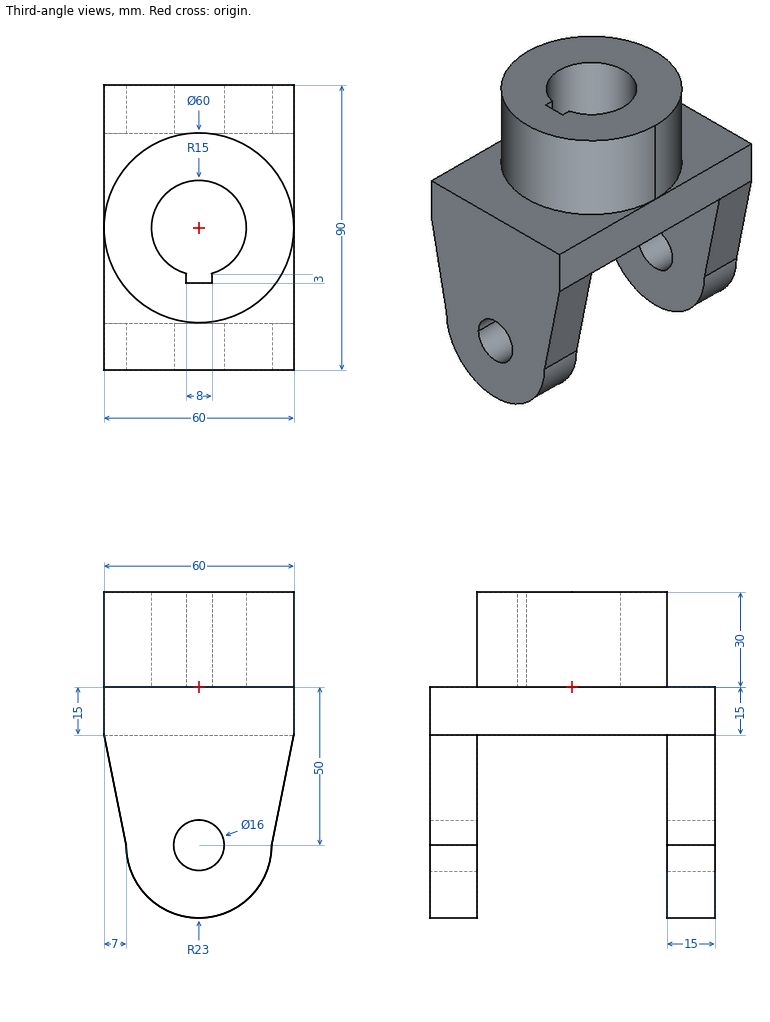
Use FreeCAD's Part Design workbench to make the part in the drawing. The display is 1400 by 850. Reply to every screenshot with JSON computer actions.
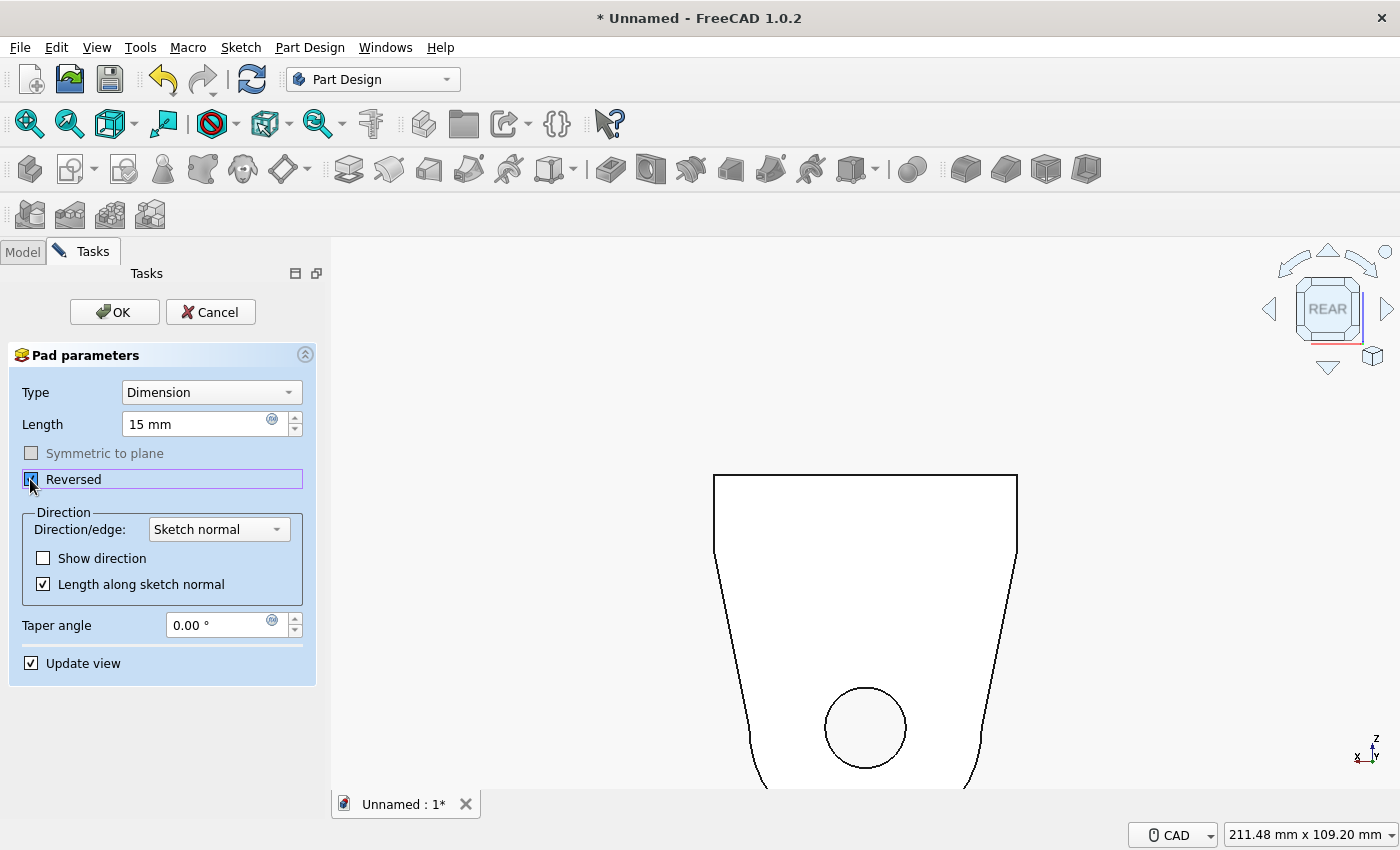
{"action": "left_click", "coordinate": [115, 312]}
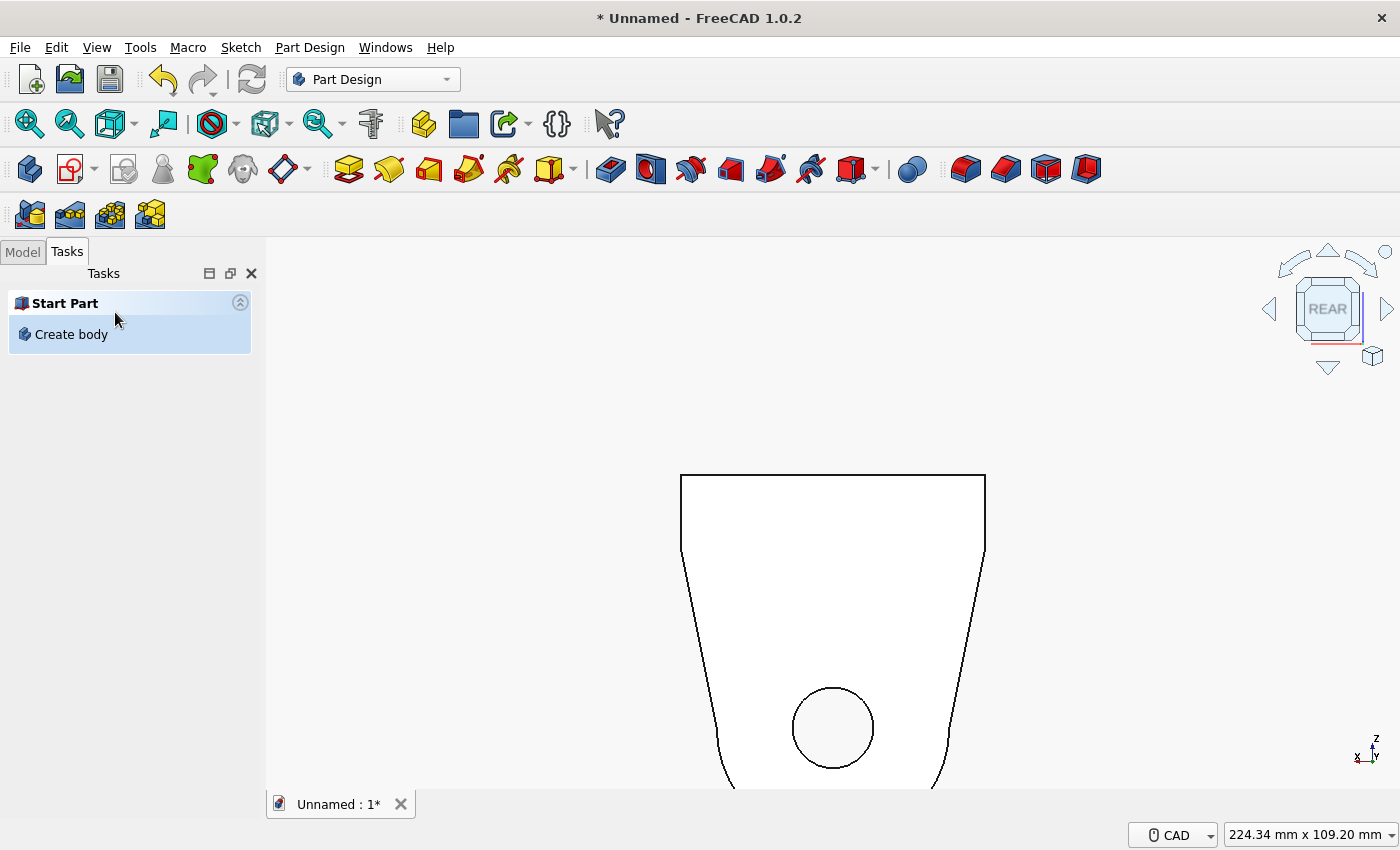
{"action": "left_click", "coordinate": [30, 124]}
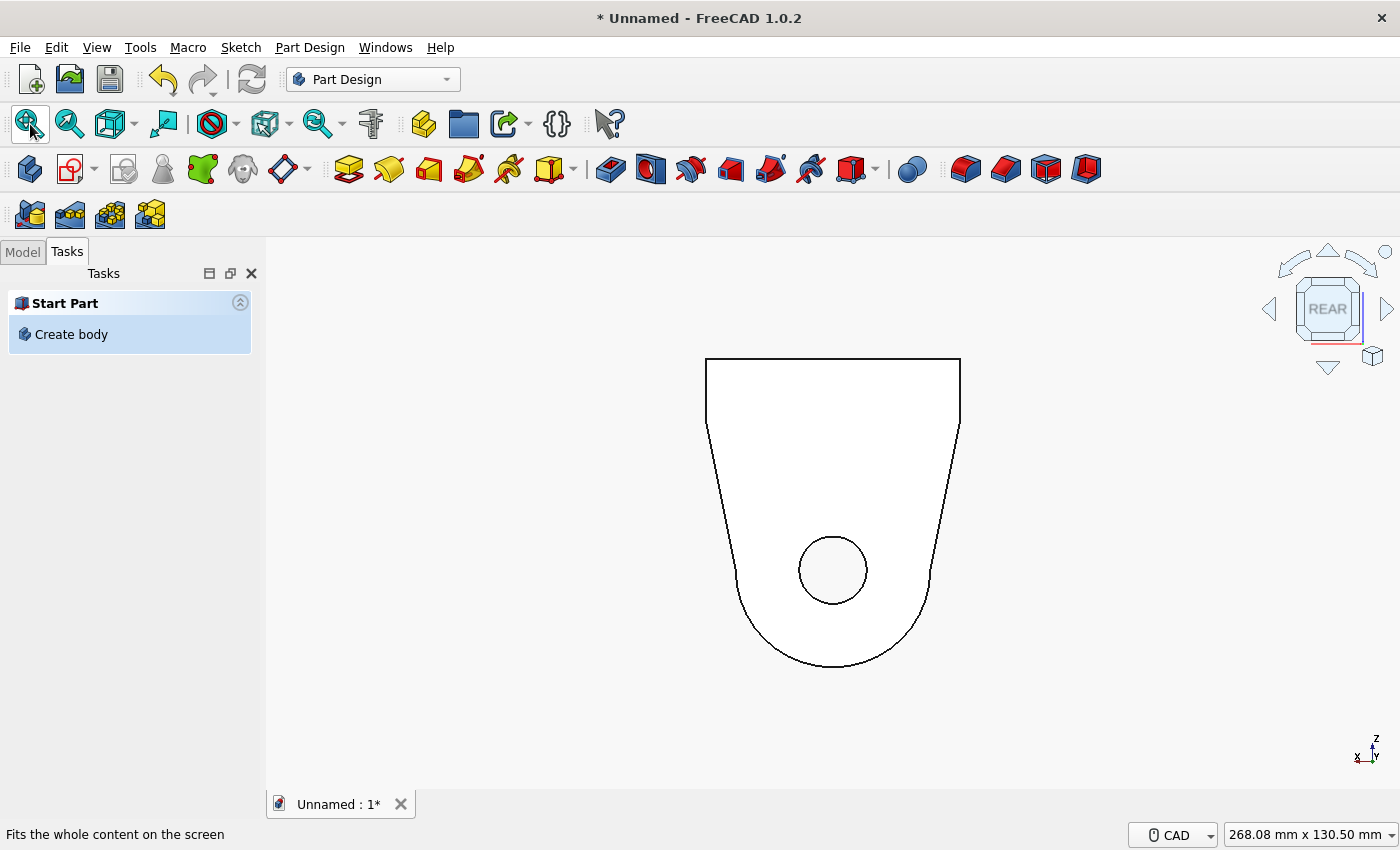
{"action": "left_click", "coordinate": [23, 251]}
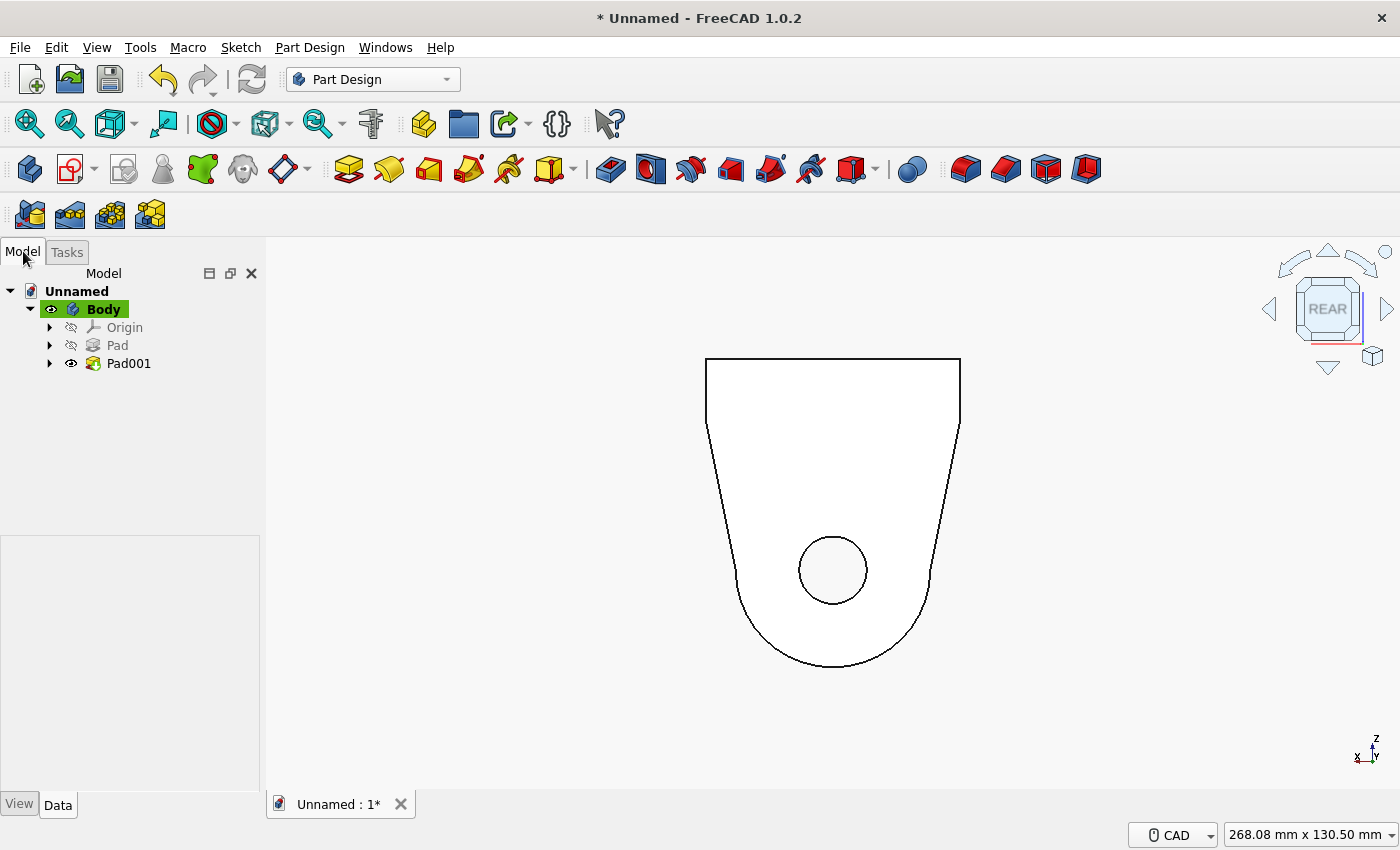
{"action": "left_click", "coordinate": [116, 363]}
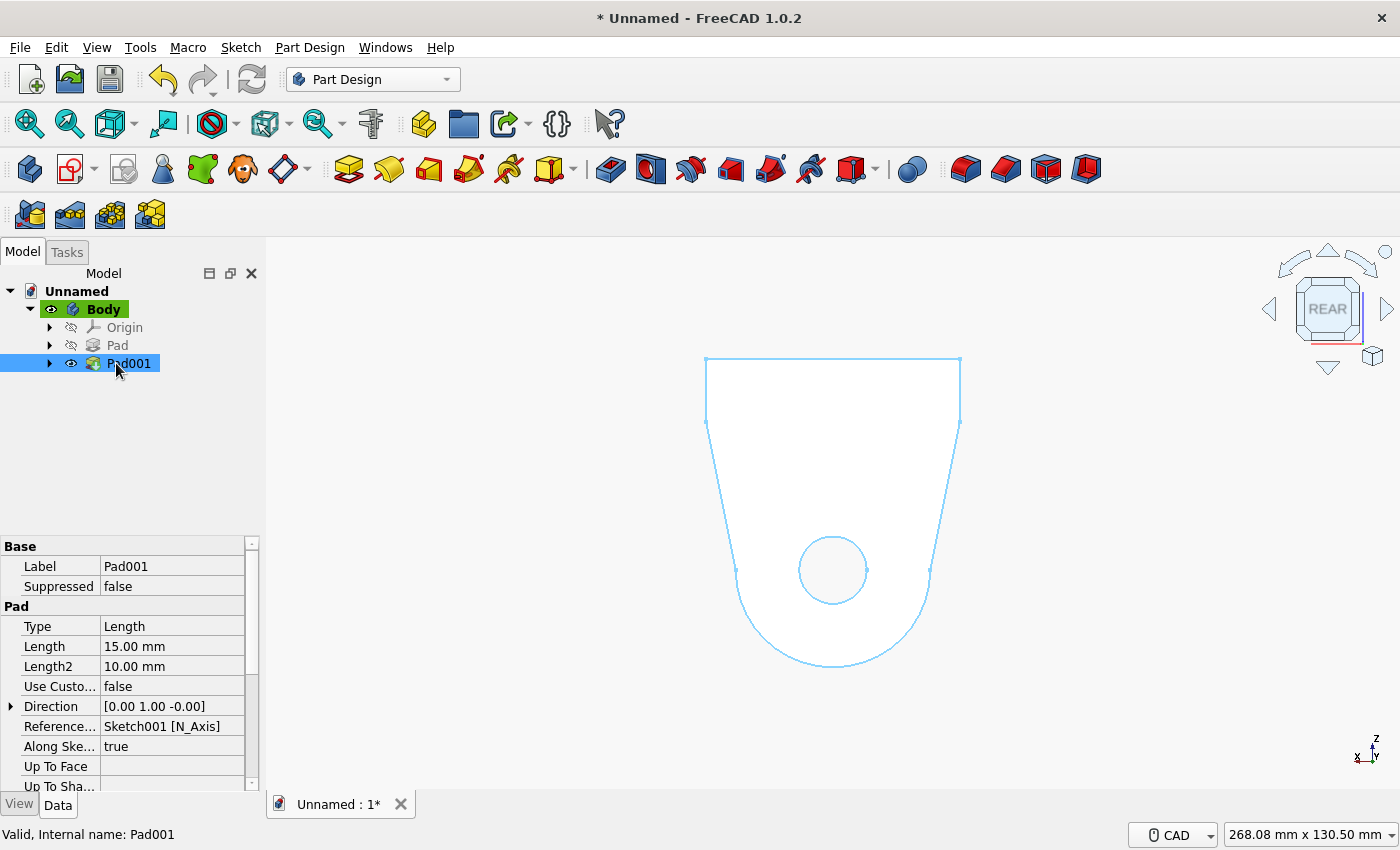
{"action": "left_click", "coordinate": [30, 214]}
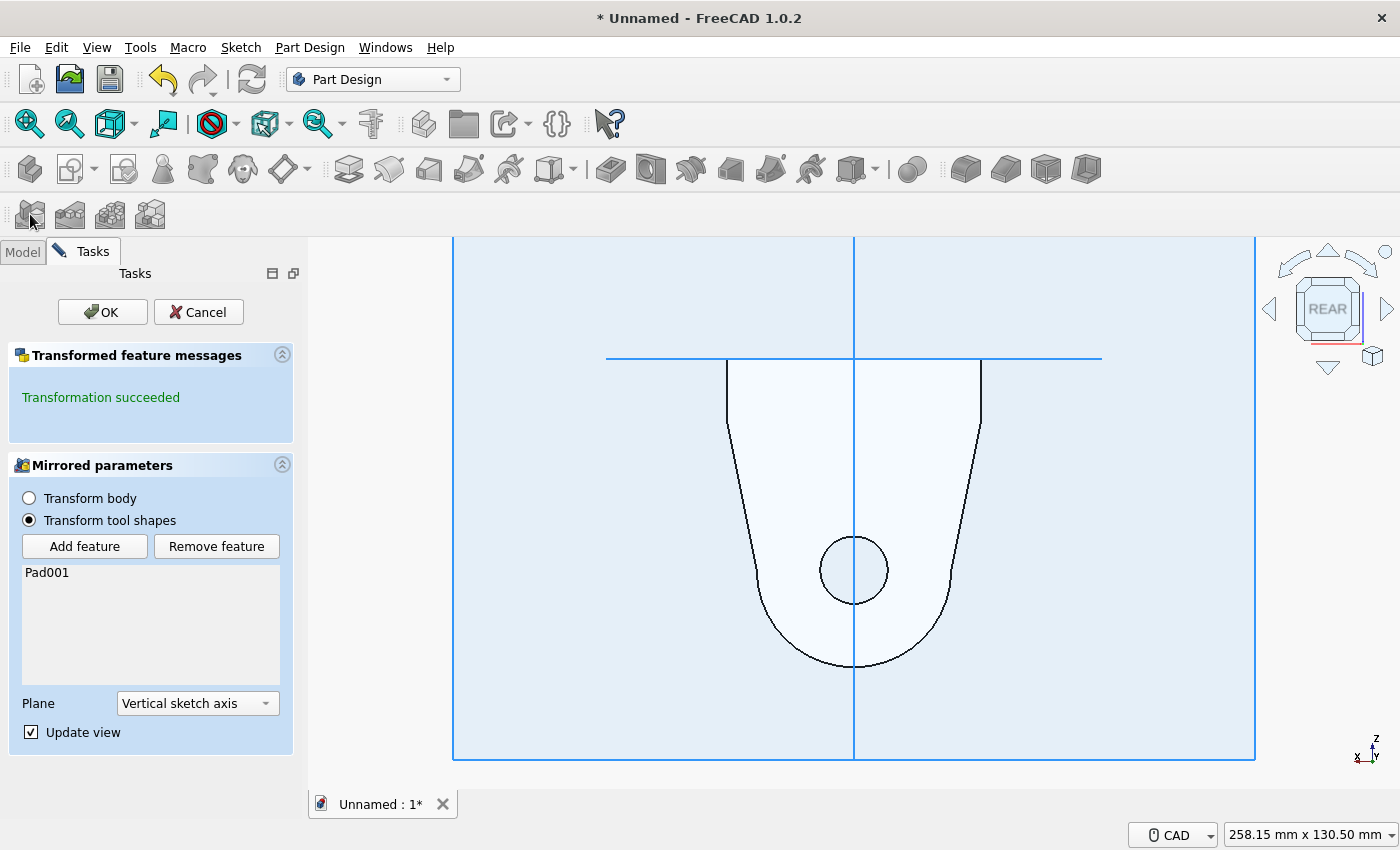
{"action": "left_click", "coordinate": [198, 704]}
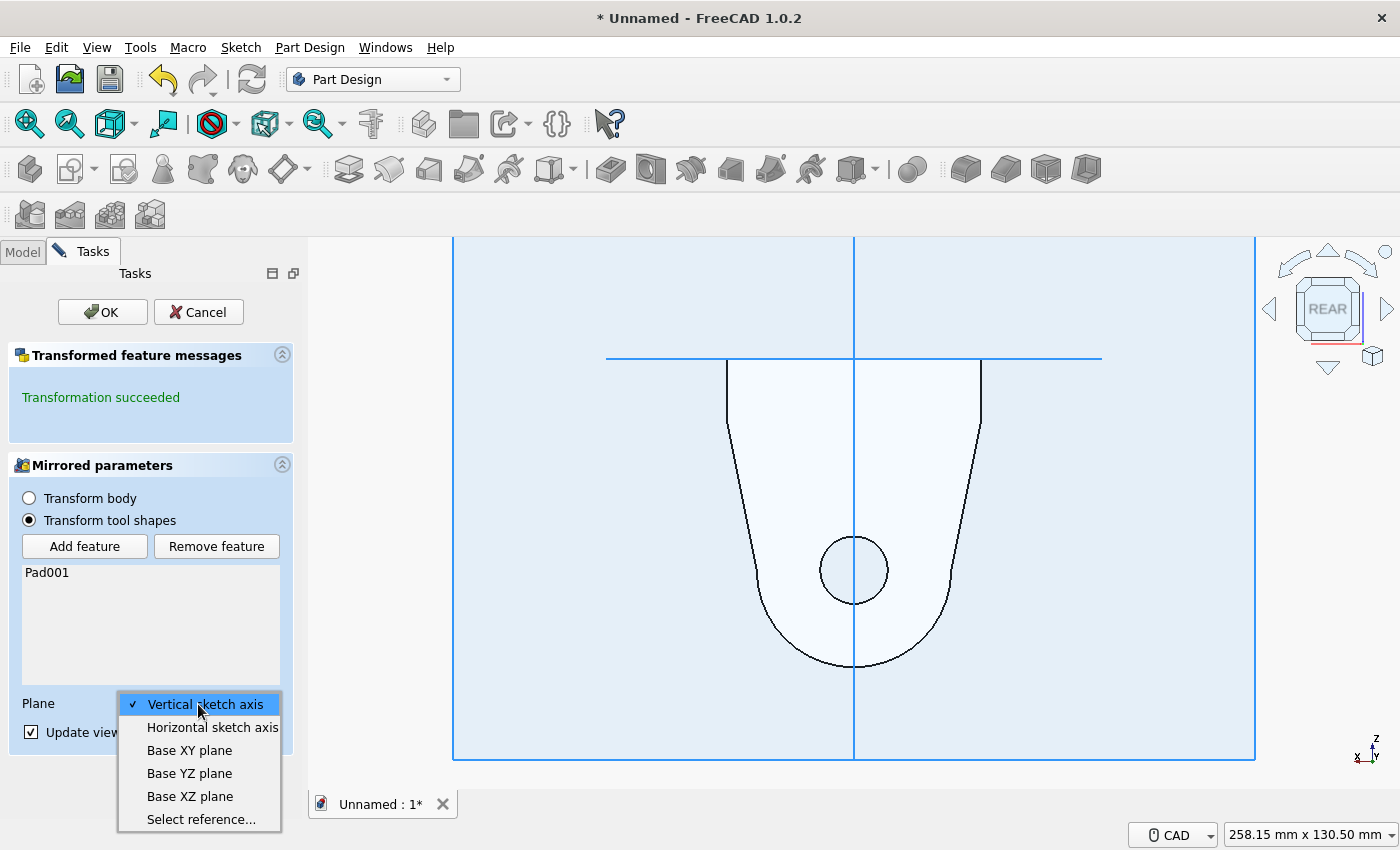
{"action": "left_click", "coordinate": [198, 796]}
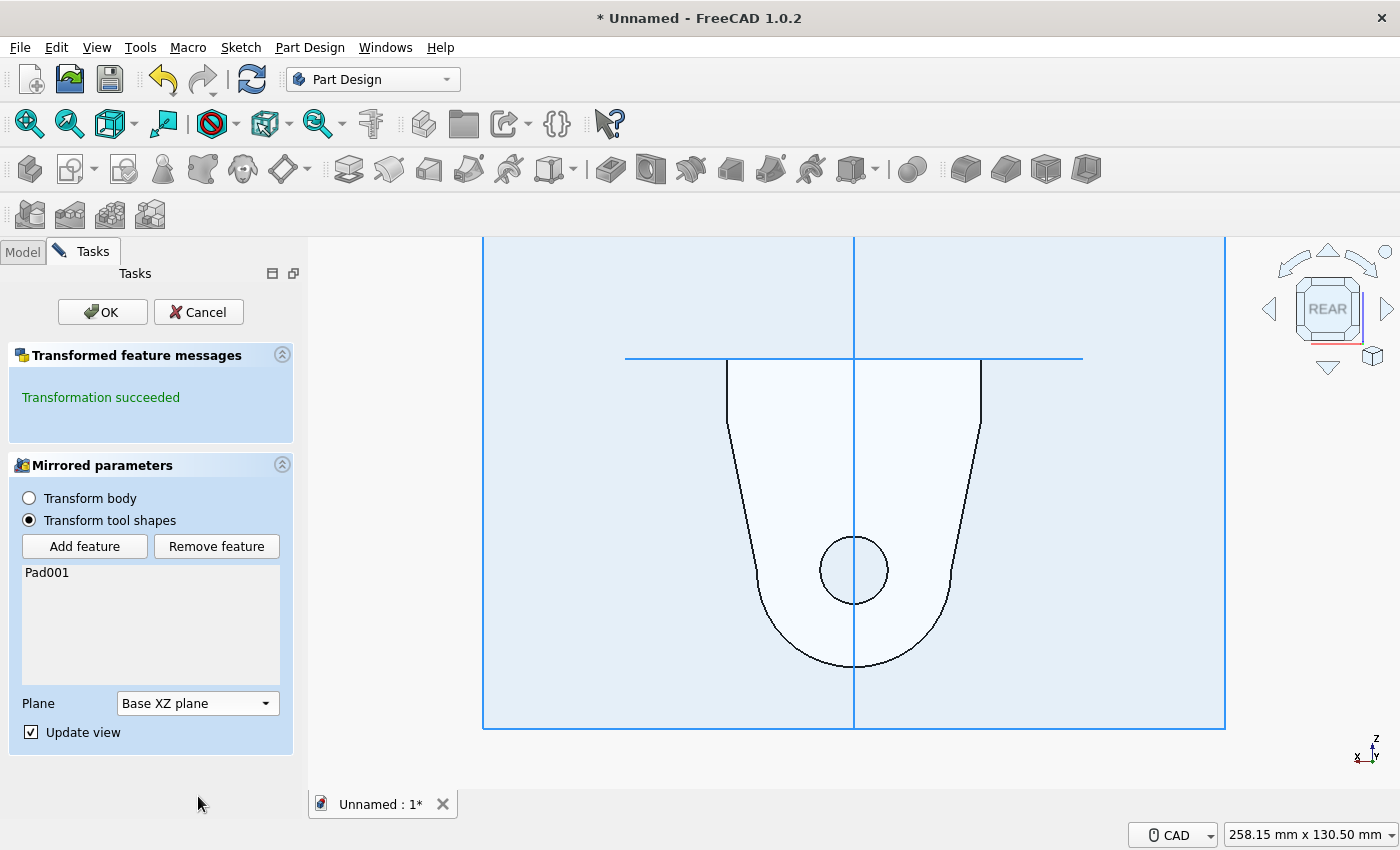
{"action": "left_click", "coordinate": [103, 312]}